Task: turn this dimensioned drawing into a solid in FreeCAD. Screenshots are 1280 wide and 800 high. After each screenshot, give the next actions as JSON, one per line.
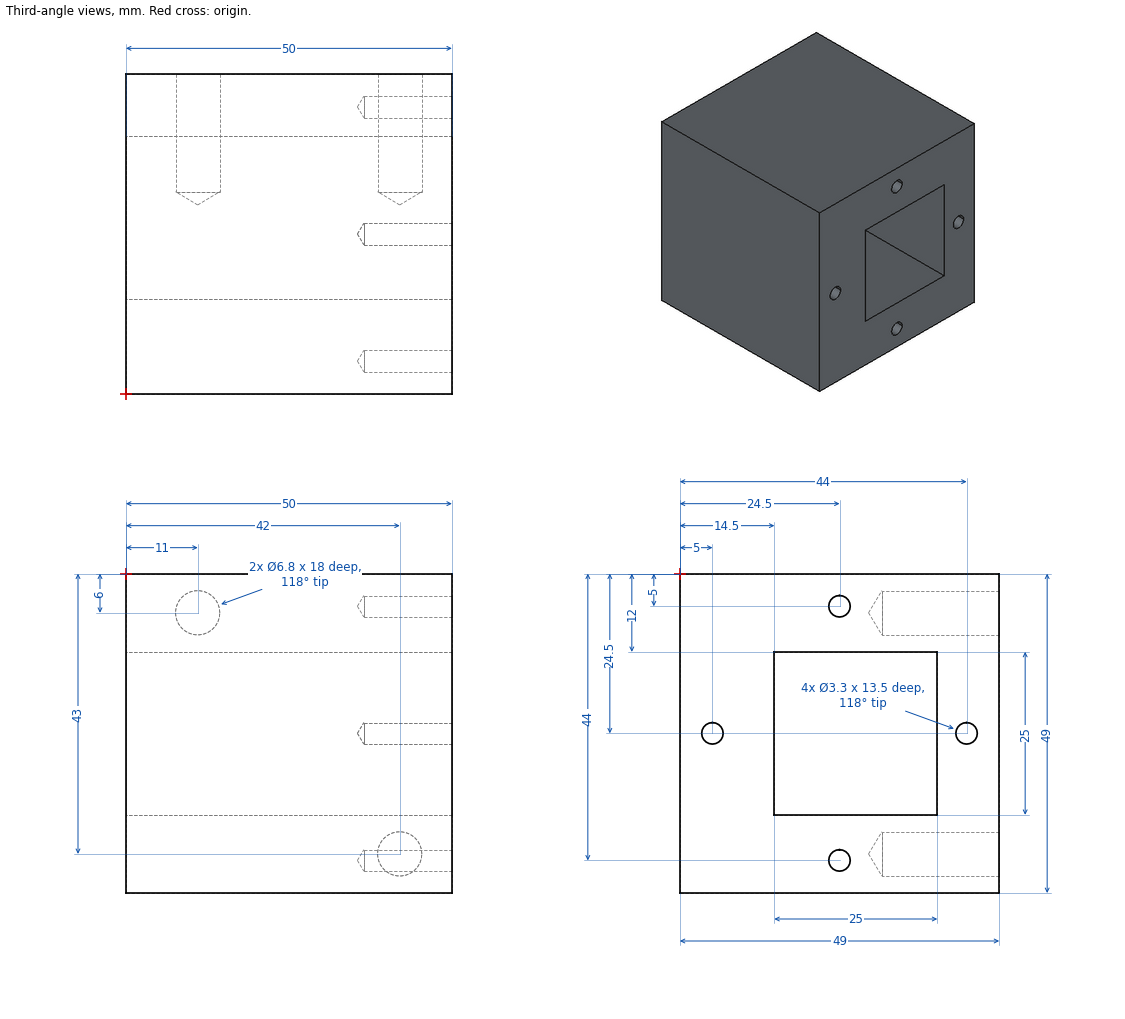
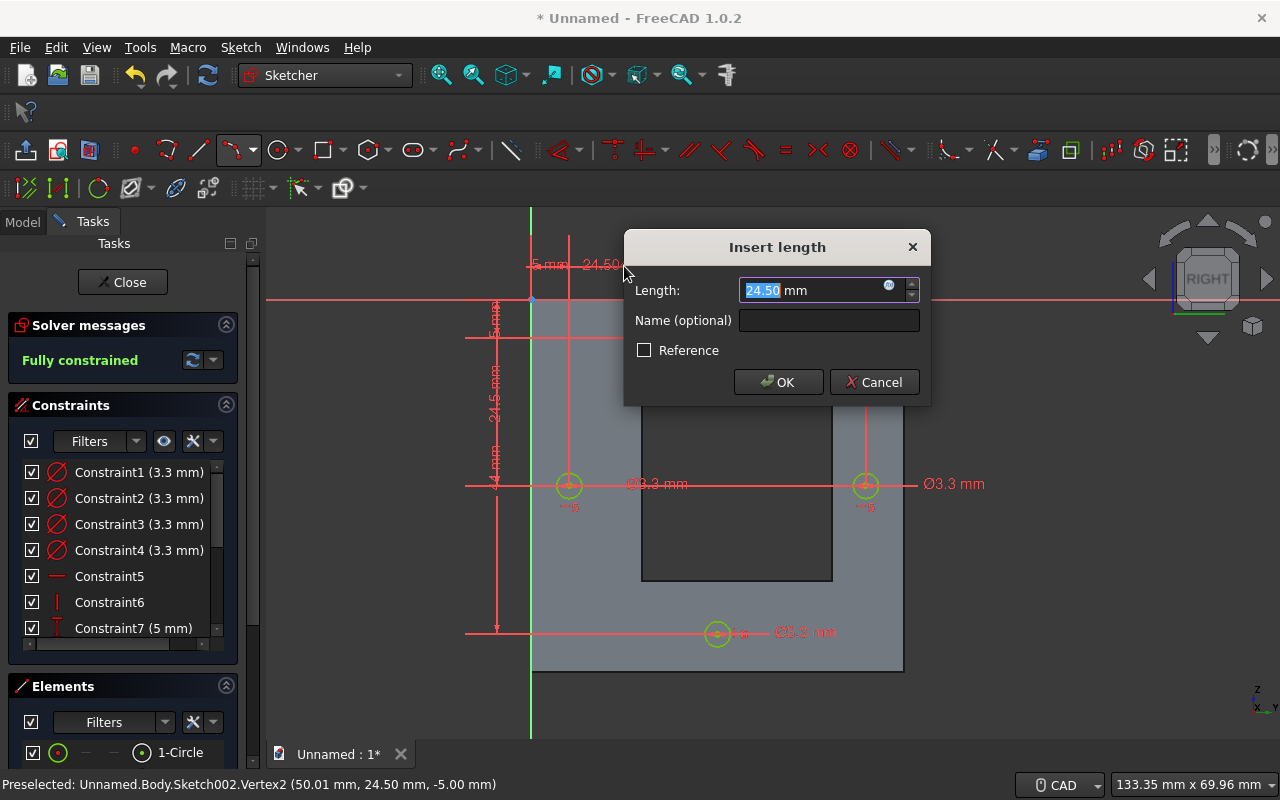
{"action": "type", "text": "24.5"}
{"action": "key", "text": "Return"}
{"action": "key", "text": "Escape"}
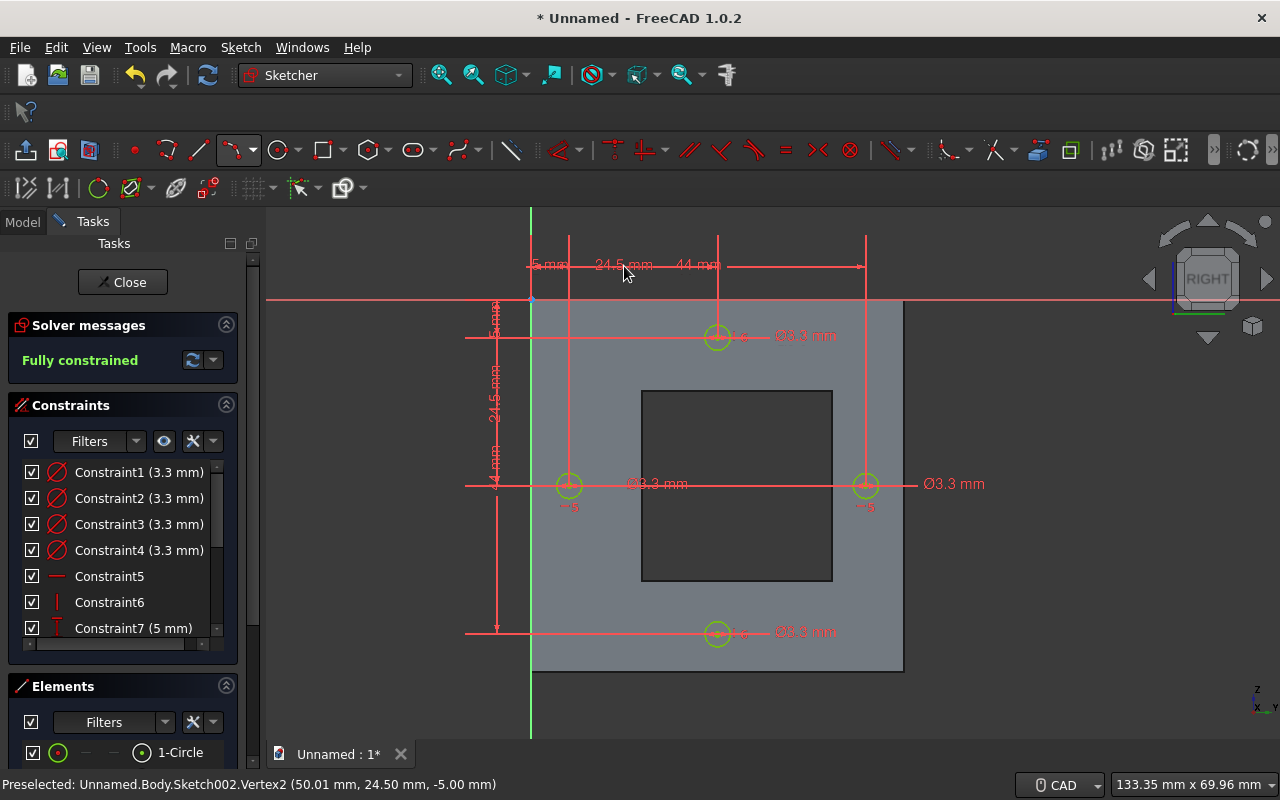
{"action": "left_click", "coordinate": [123, 282]}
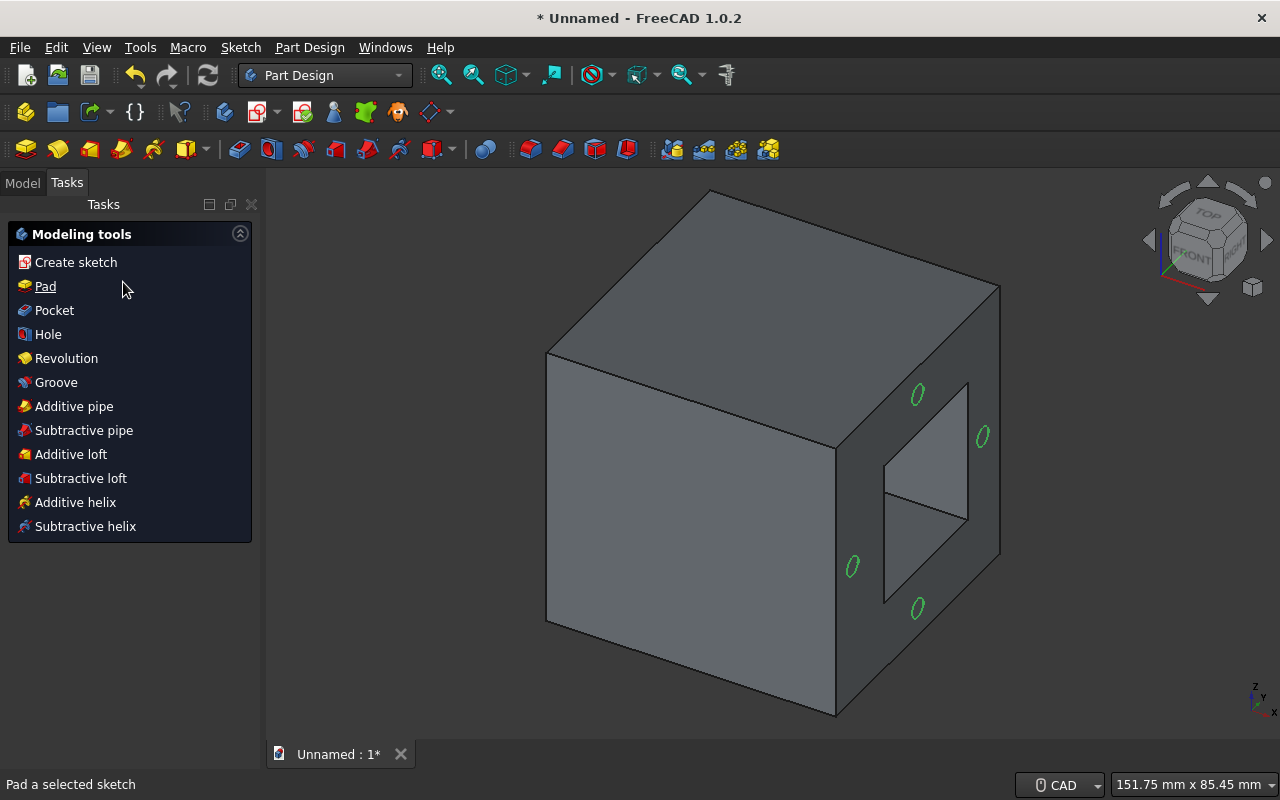
{"action": "left_click", "coordinate": [272, 150]}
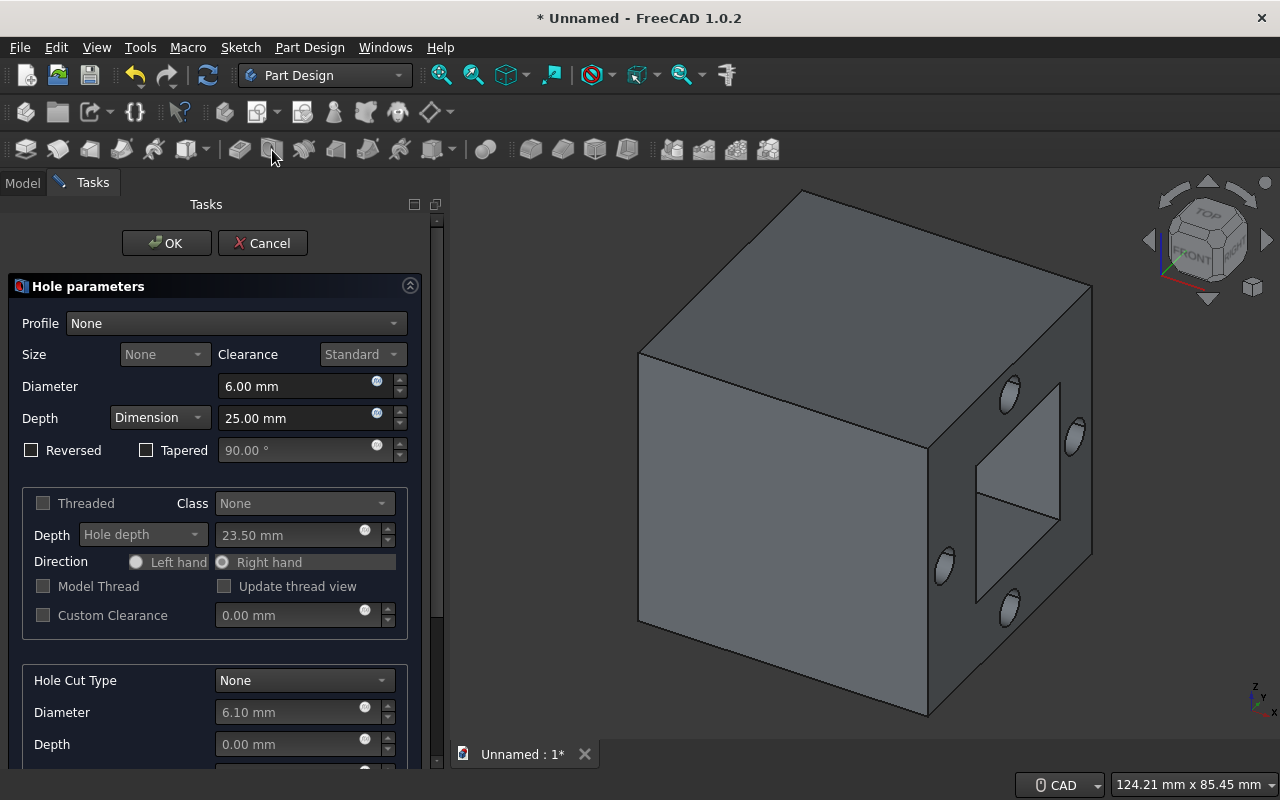
{"action": "triple_click", "coordinate": [305, 386]}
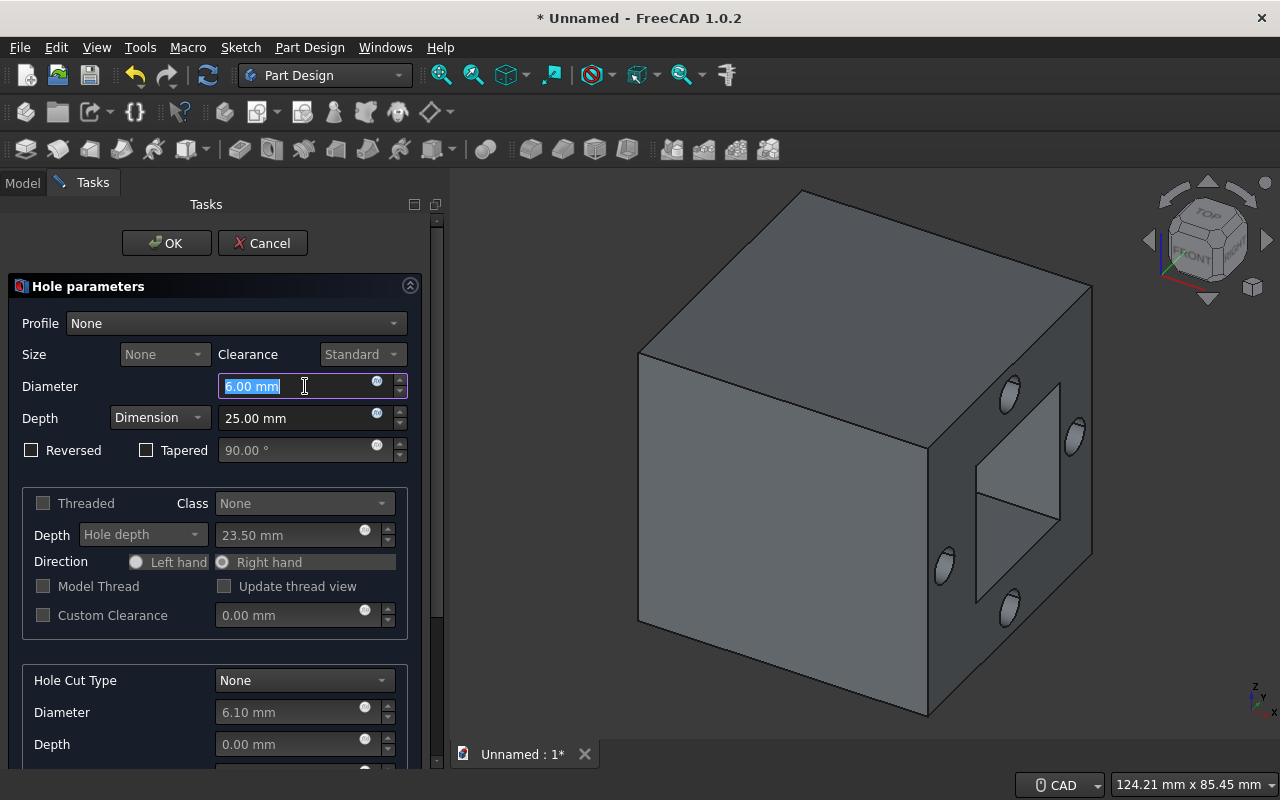
{"action": "type", "text": "3.3"}
{"action": "key", "text": "Tab"}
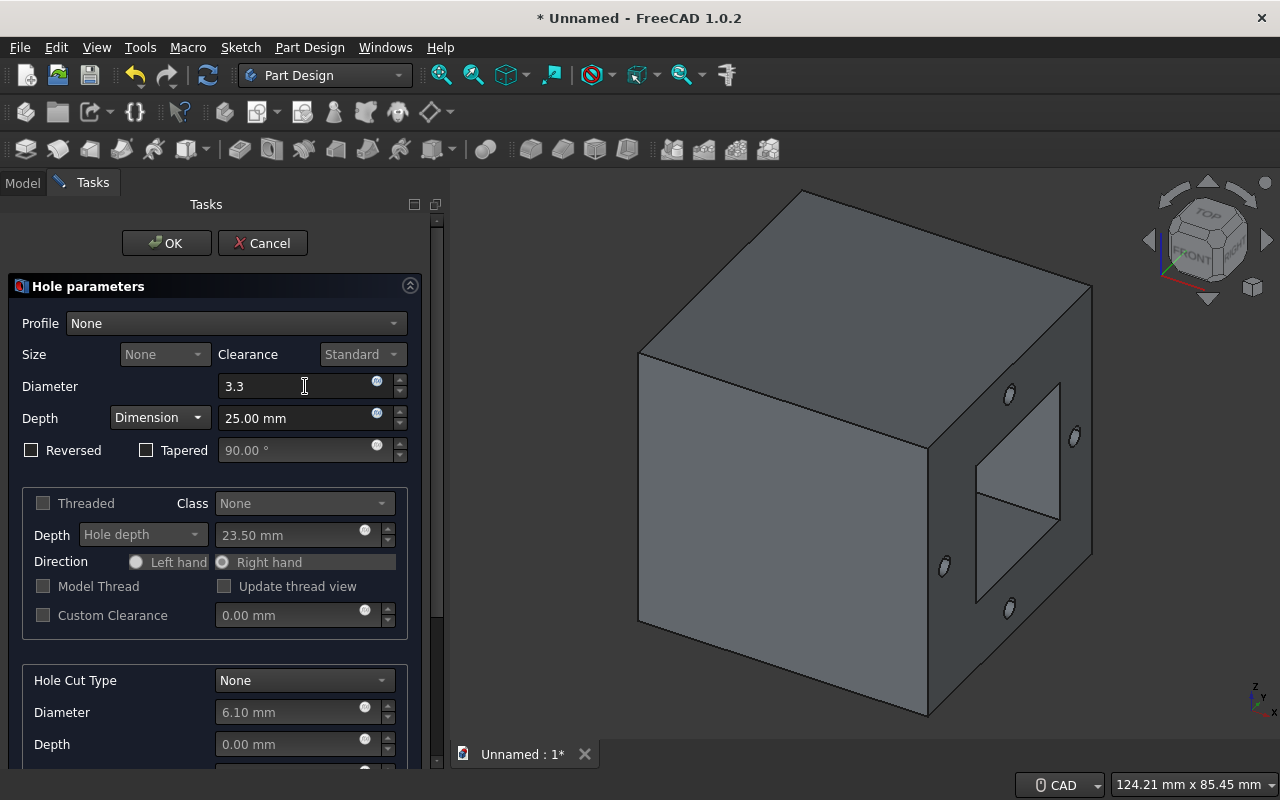
{"action": "triple_click", "coordinate": [305, 418]}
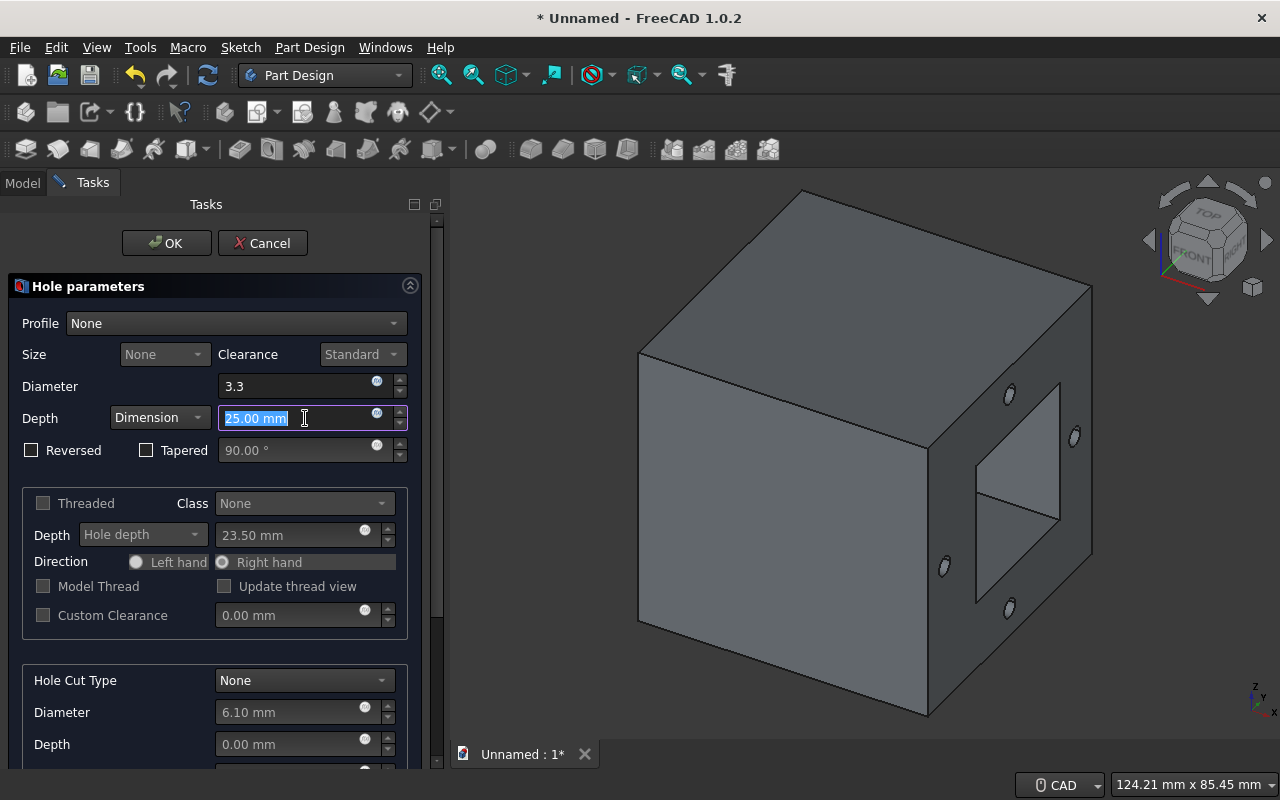
{"action": "type", "text": "13.5"}
{"action": "key", "text": "Tab"}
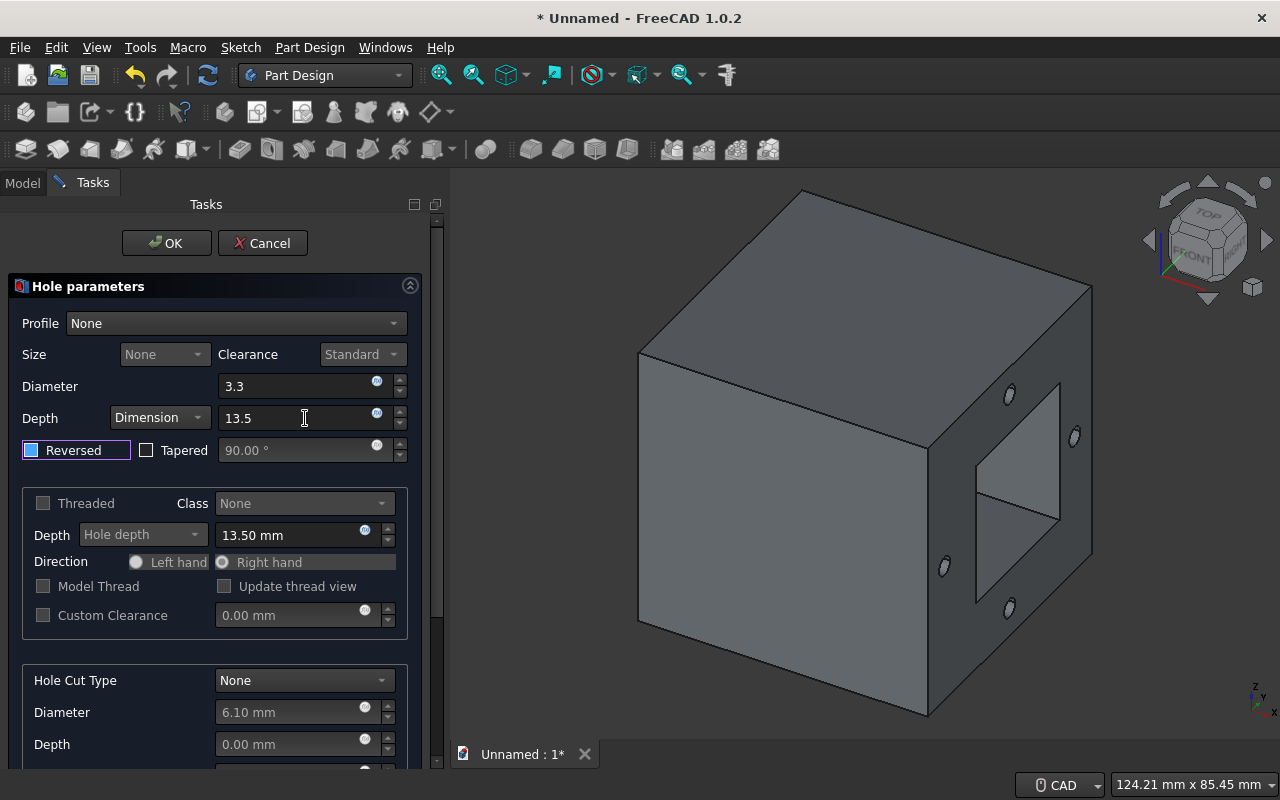
{"action": "left_click", "coordinate": [167, 243]}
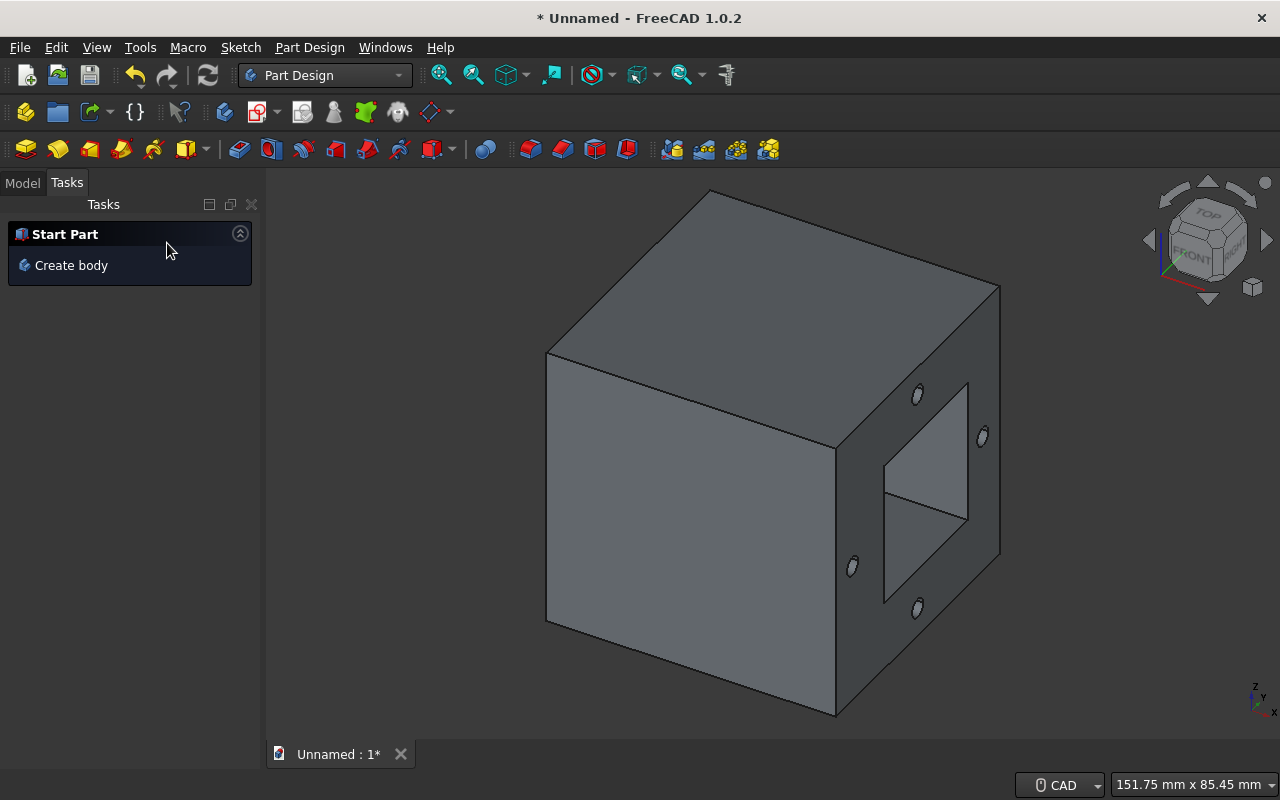
{"action": "key", "text": "4"}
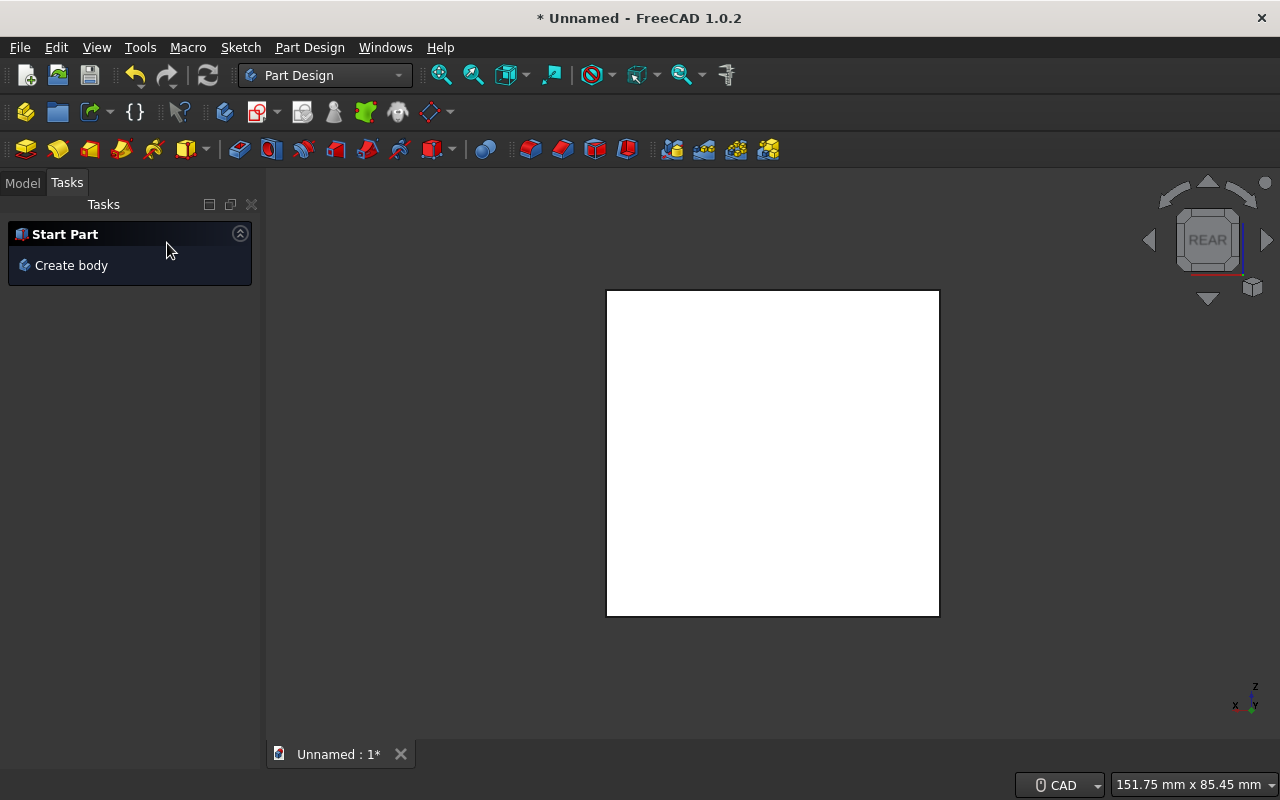
{"action": "left_click", "coordinate": [773, 452]}